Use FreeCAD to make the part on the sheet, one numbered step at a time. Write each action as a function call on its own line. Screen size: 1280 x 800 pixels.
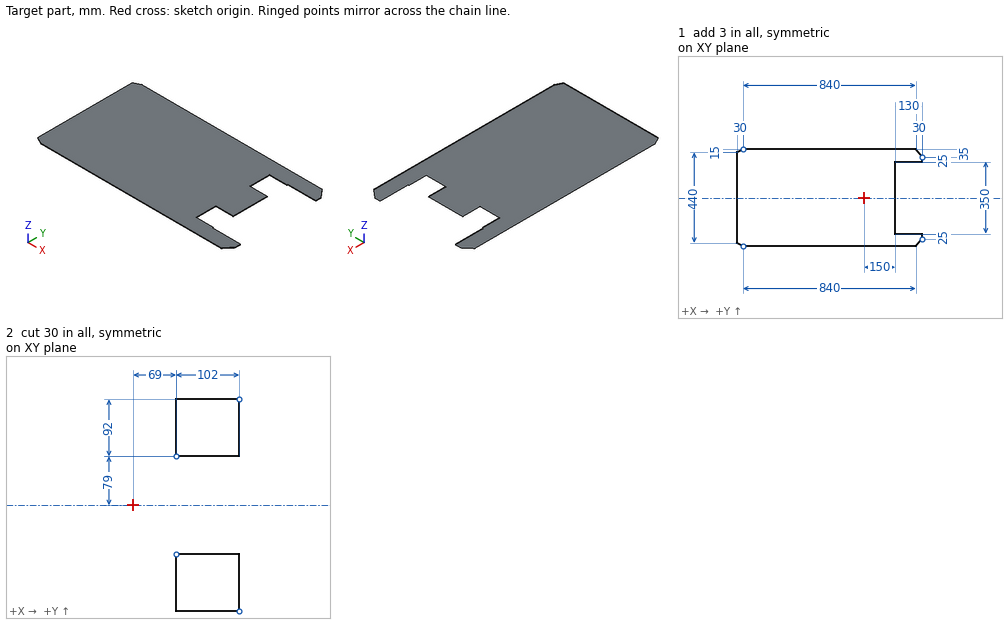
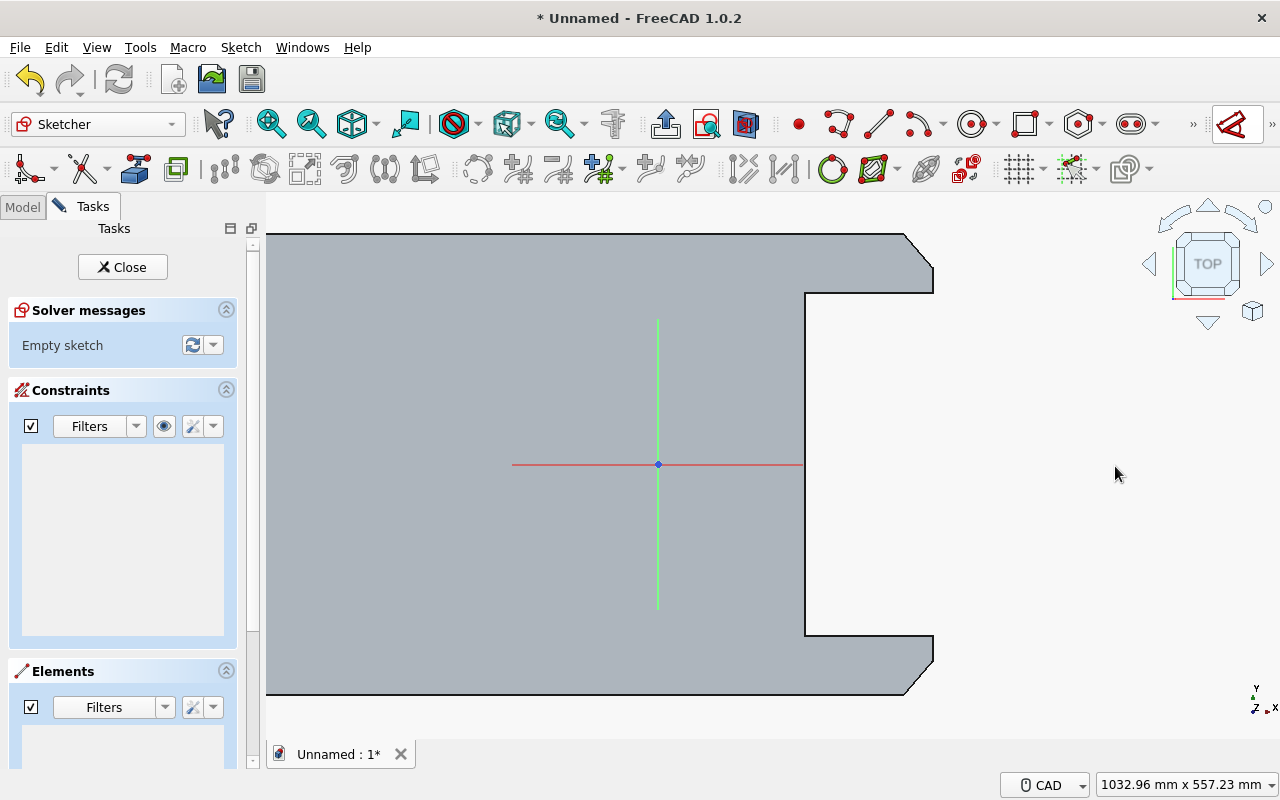
key(g)
key(r)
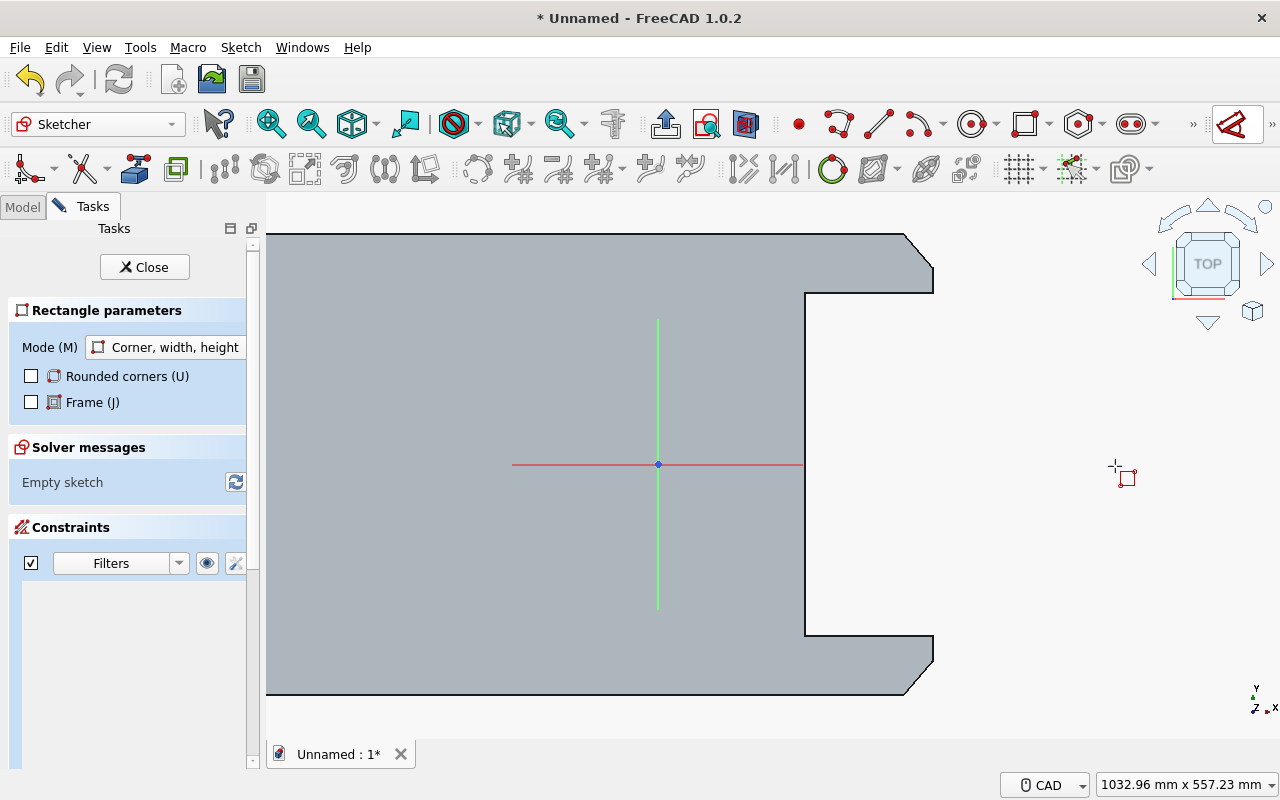
click(726, 297)
click(826, 387)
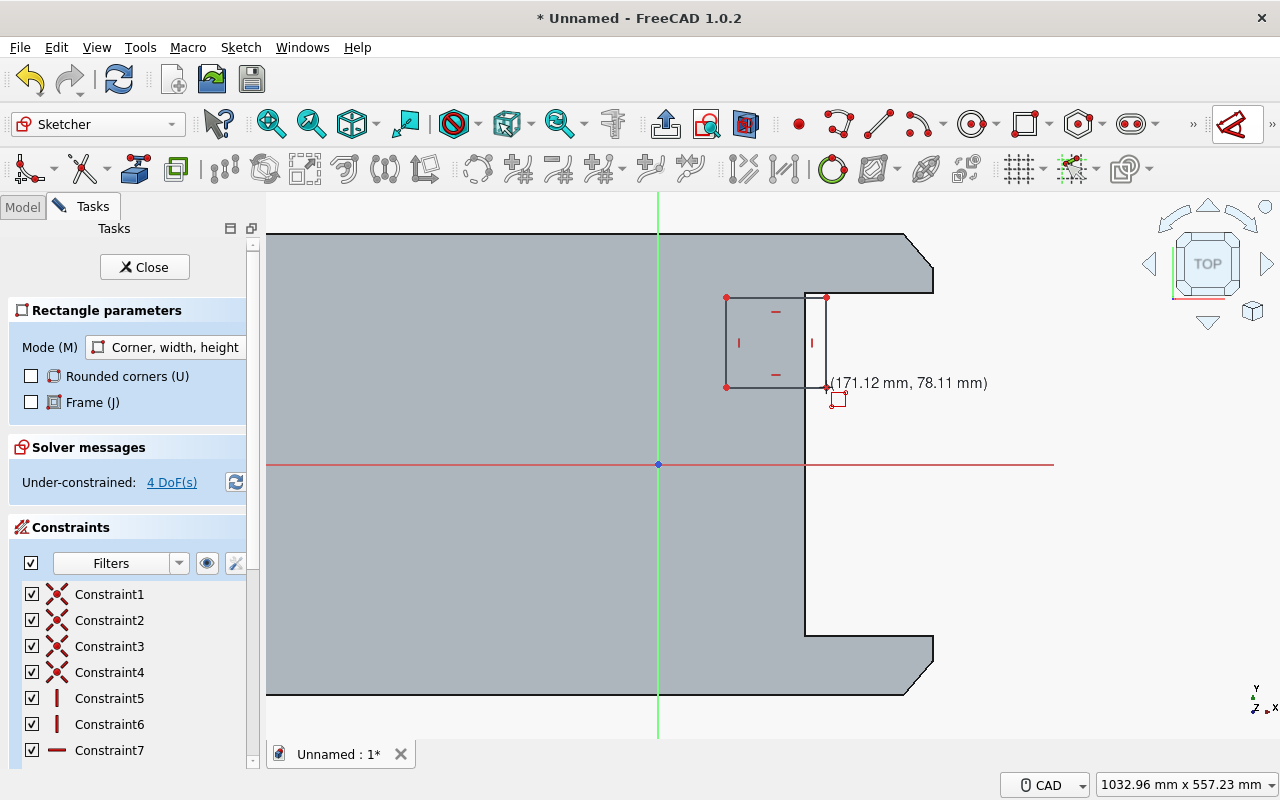
click(726, 542)
click(826, 633)
key(Escape)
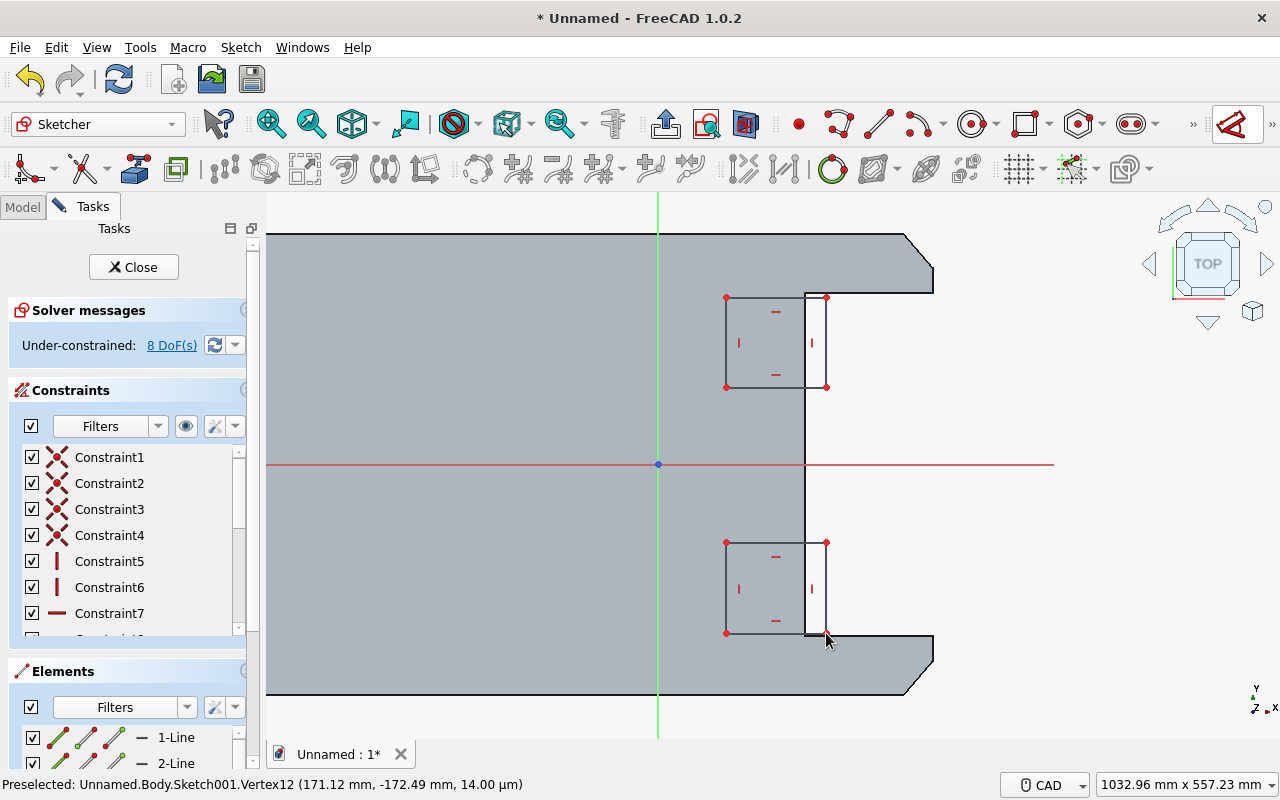
click(726, 388)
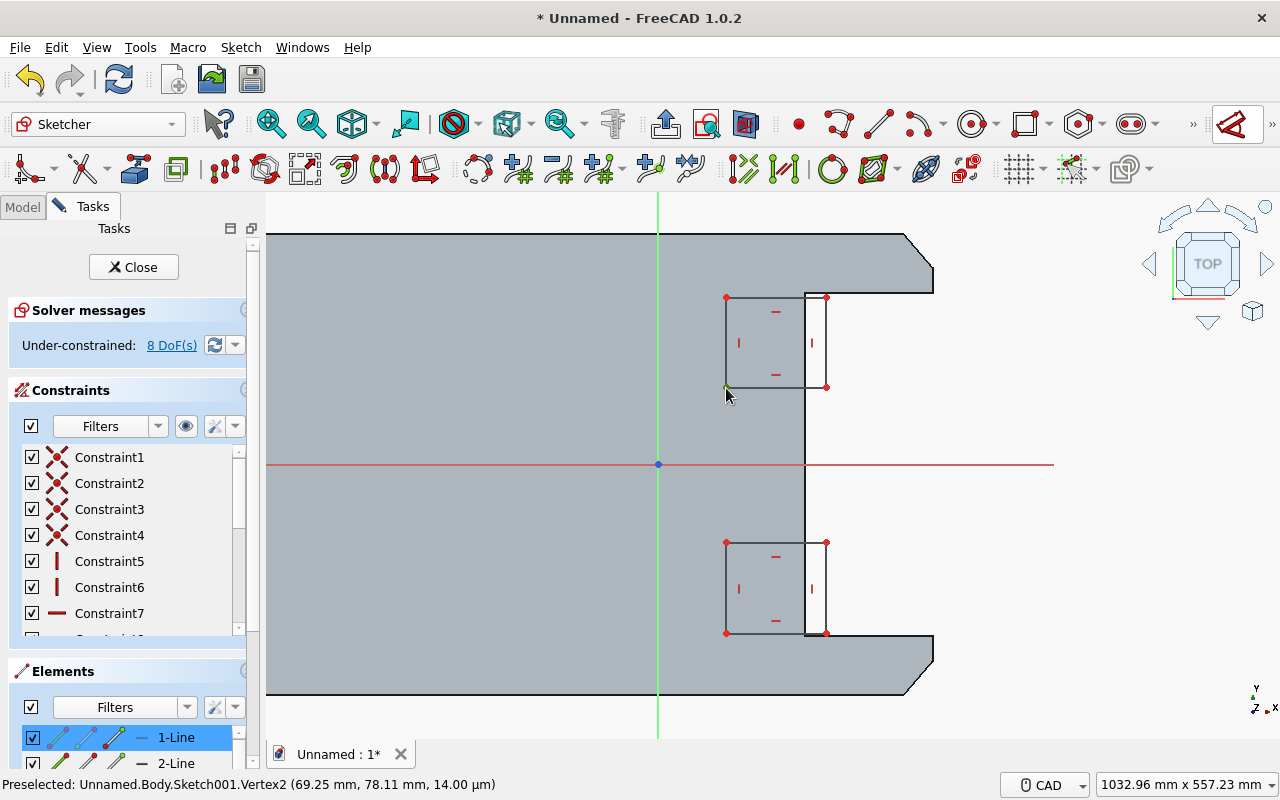
click(726, 543)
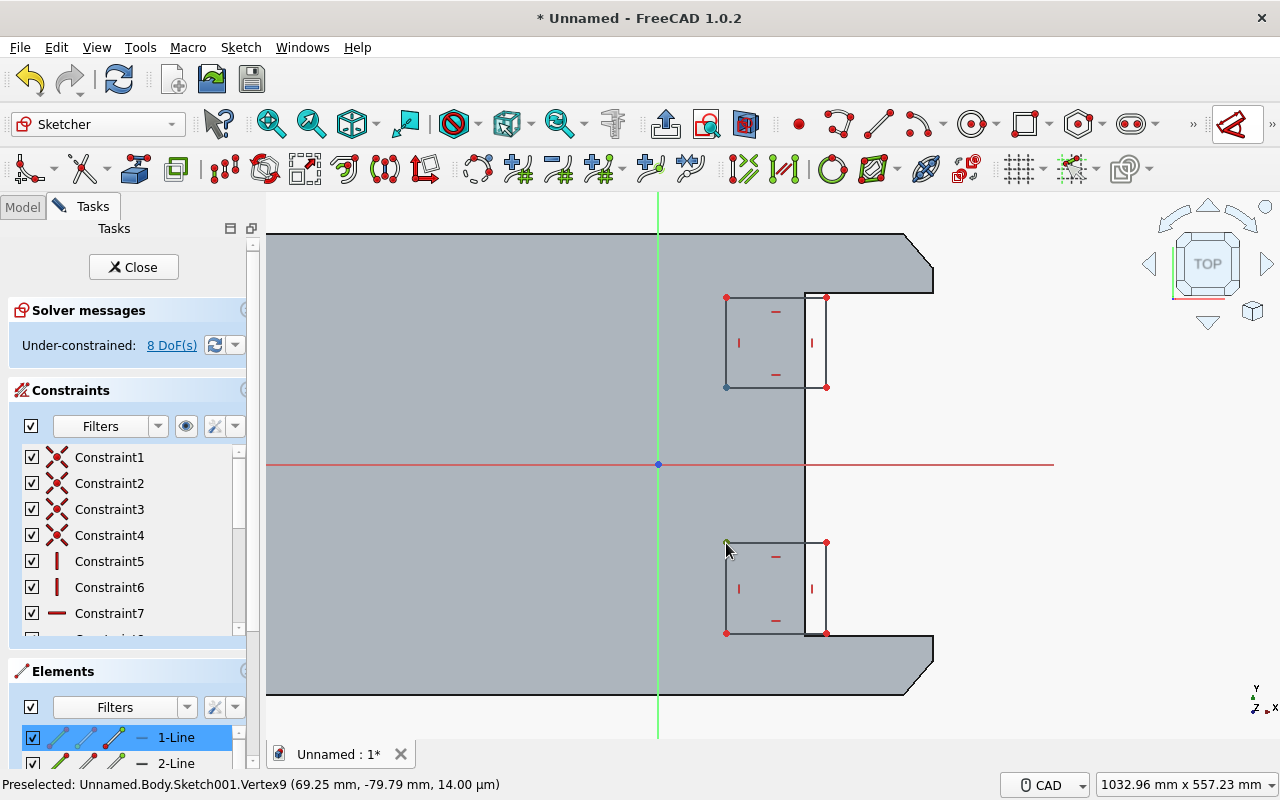
click(353, 465)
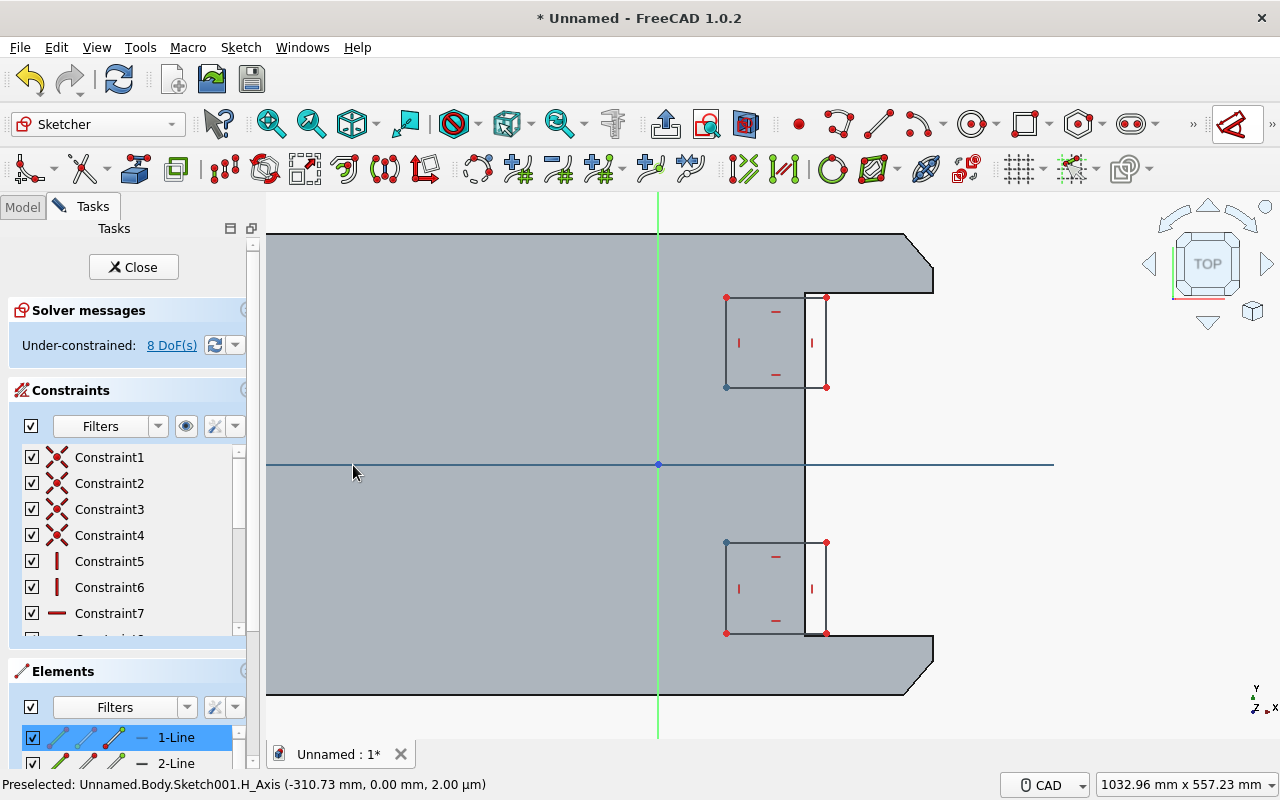
key(s)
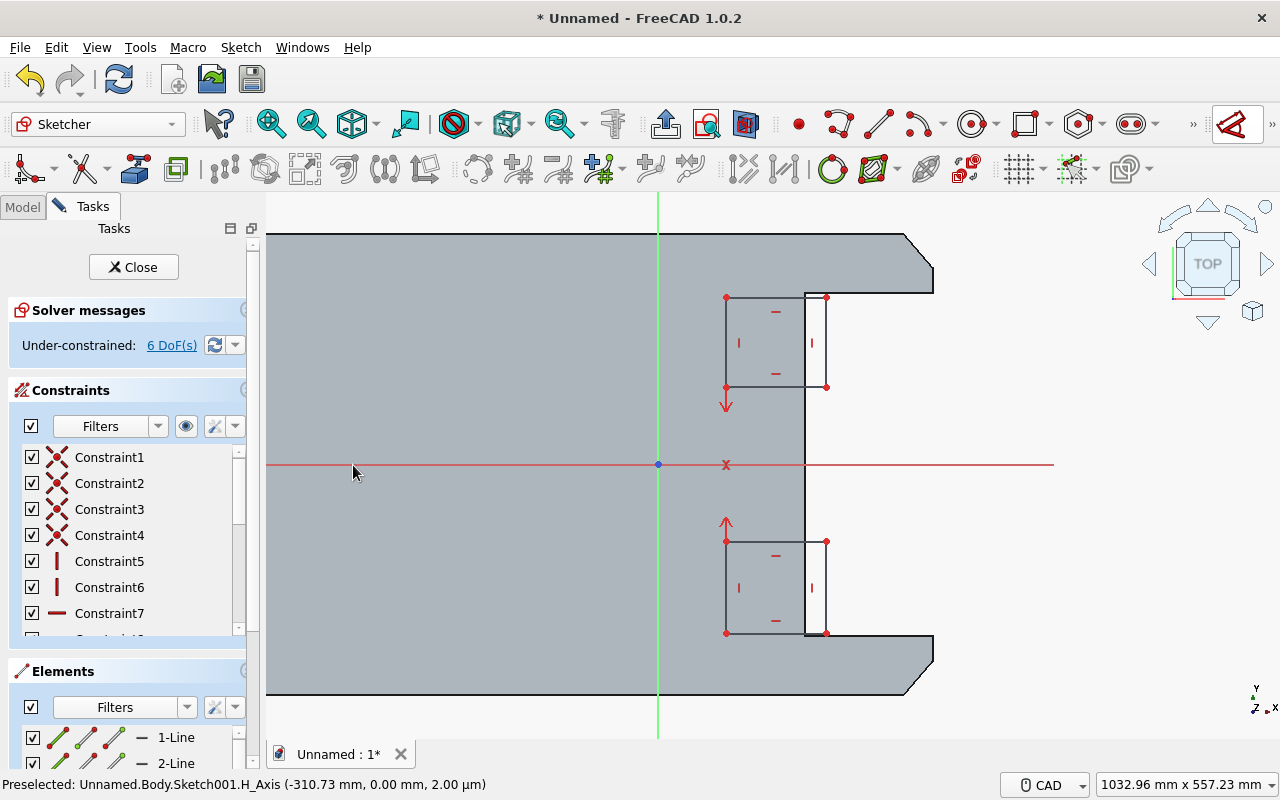
click(826, 298)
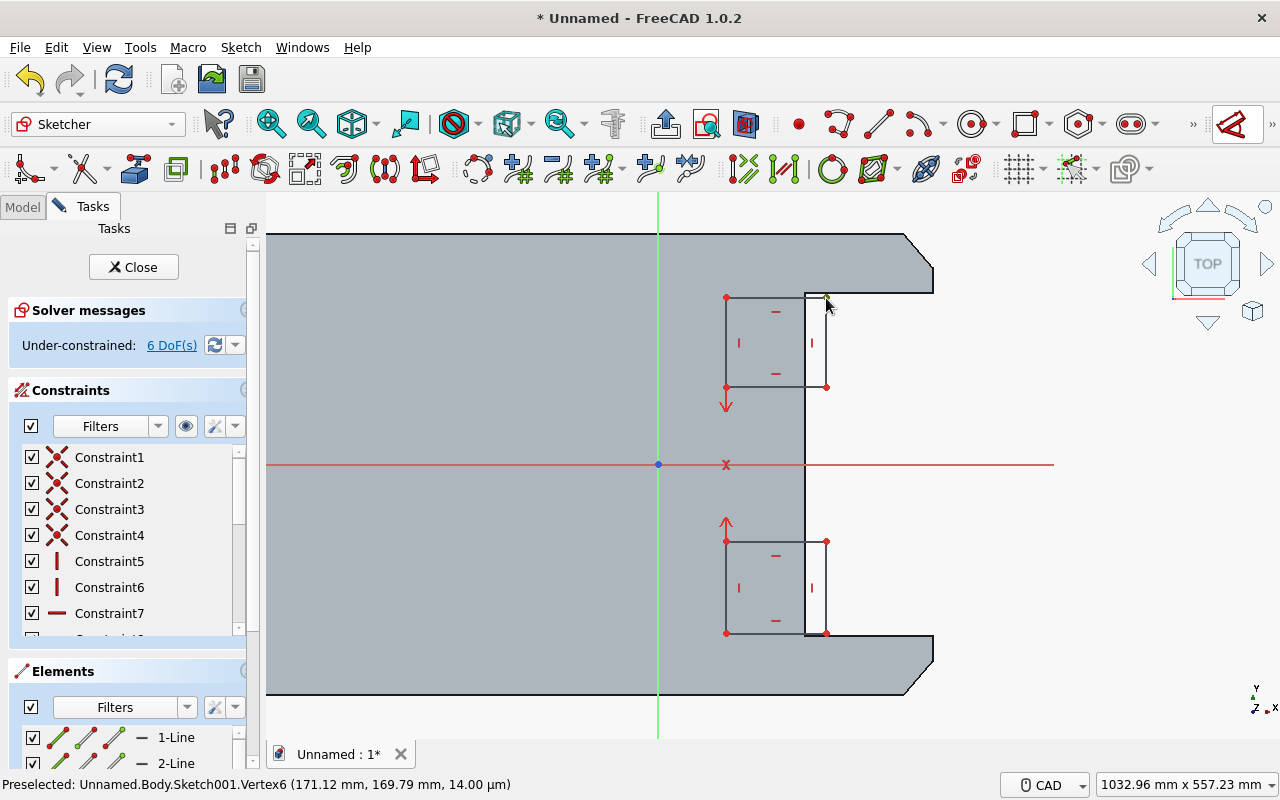
click(826, 634)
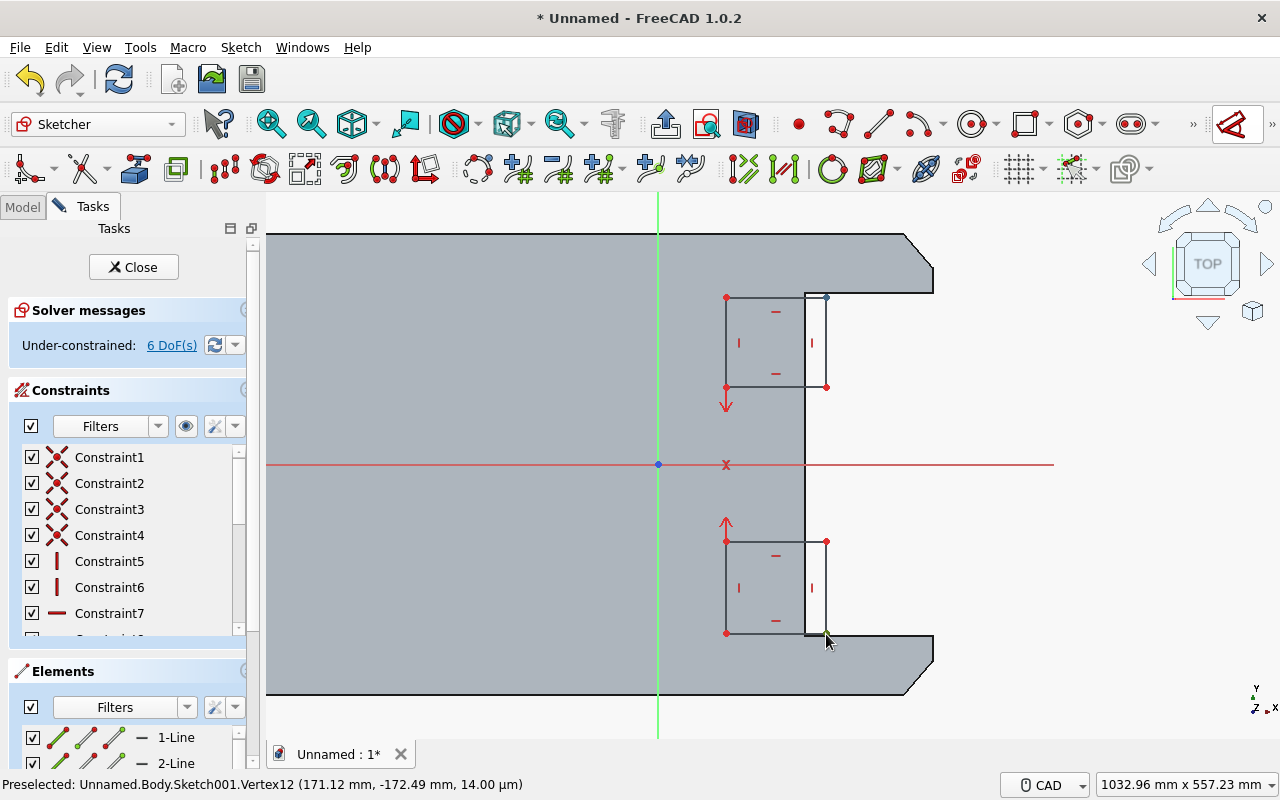
click(353, 465)